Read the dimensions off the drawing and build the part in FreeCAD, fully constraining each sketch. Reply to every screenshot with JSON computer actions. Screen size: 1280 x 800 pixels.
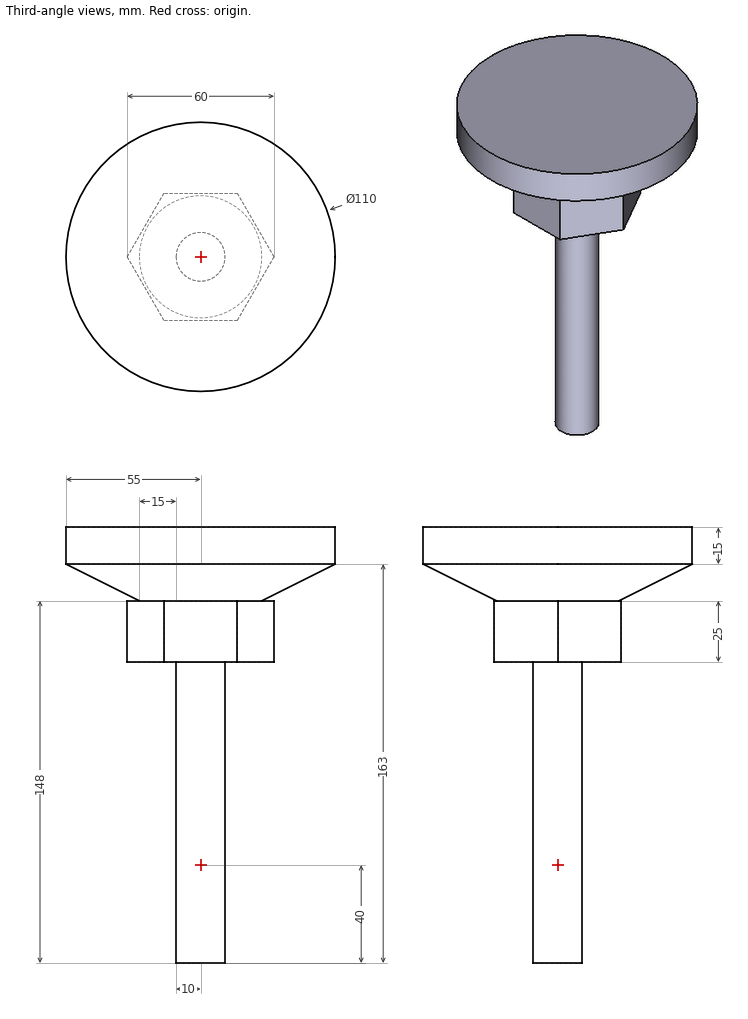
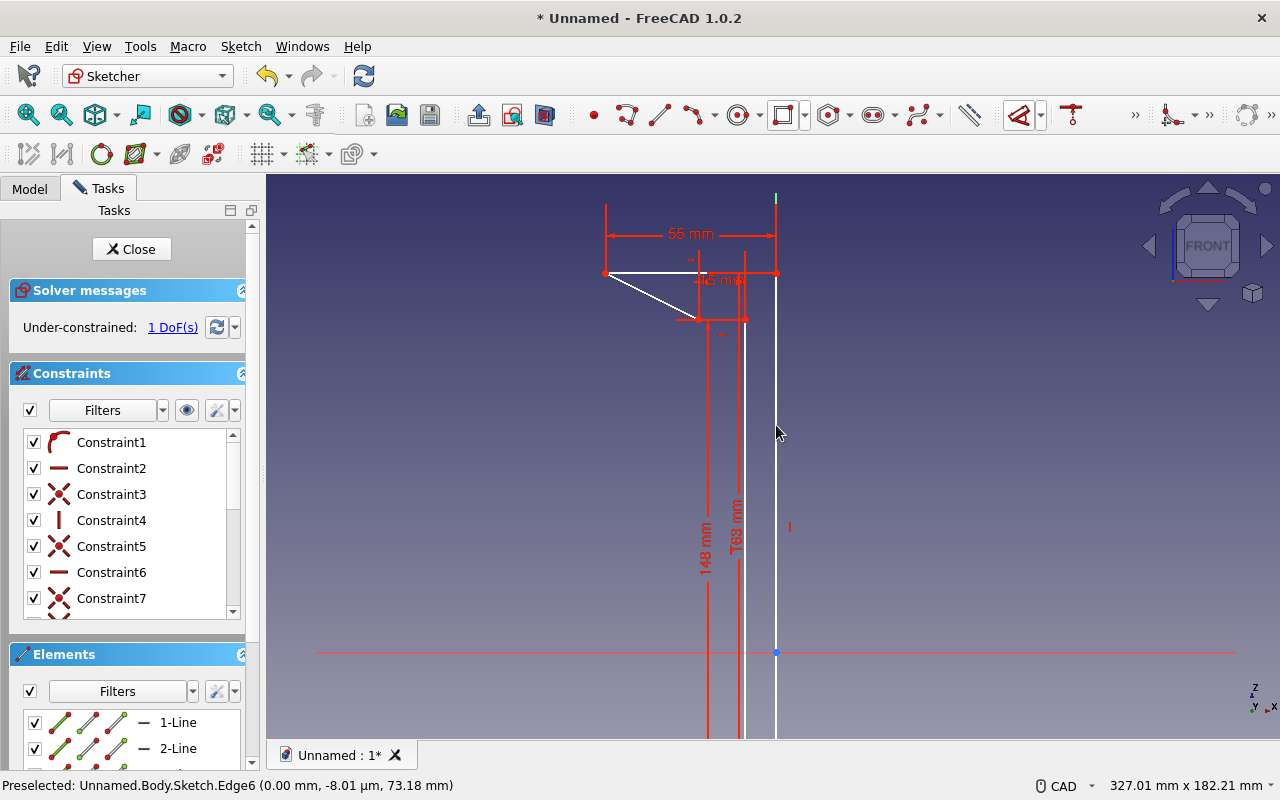
{"action": "scroll", "coordinate": [732, 319], "scroll_direction": "down", "scroll_amount": 2}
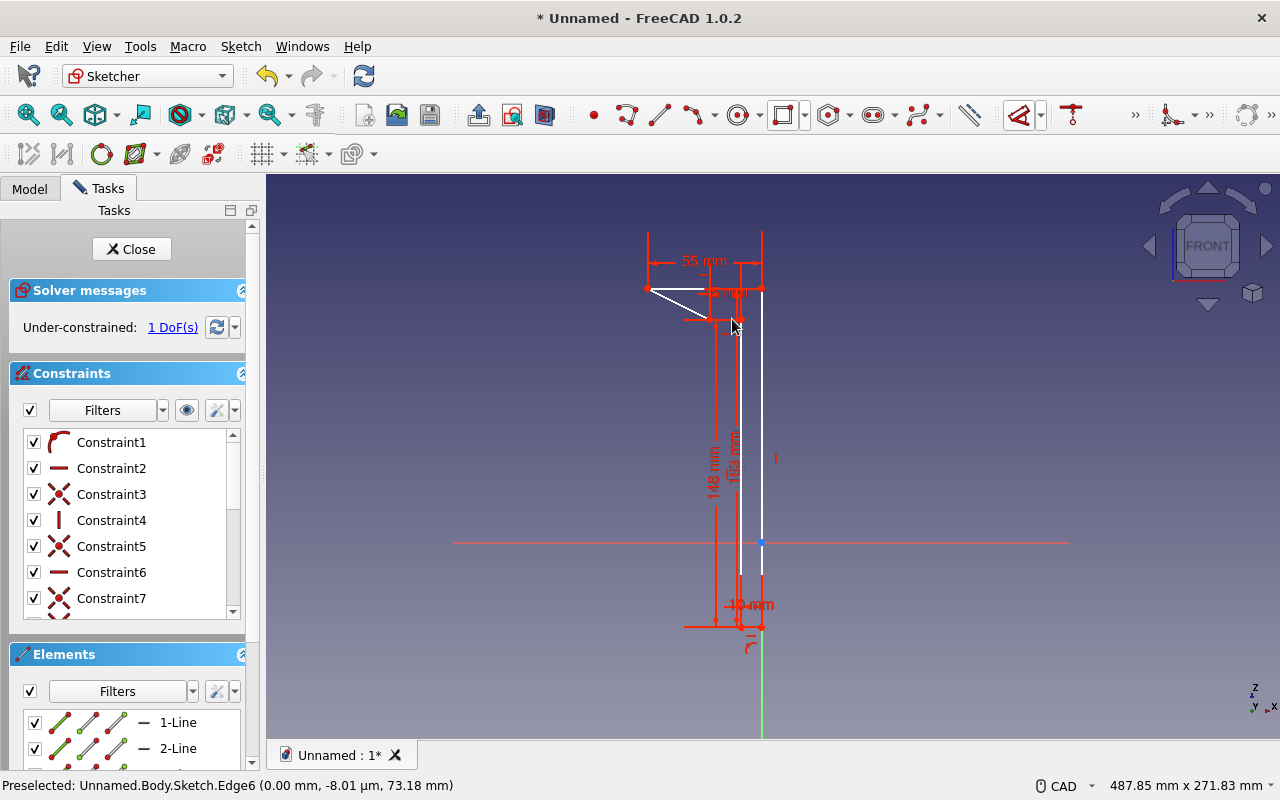
{"action": "left_click", "coordinate": [762, 627]}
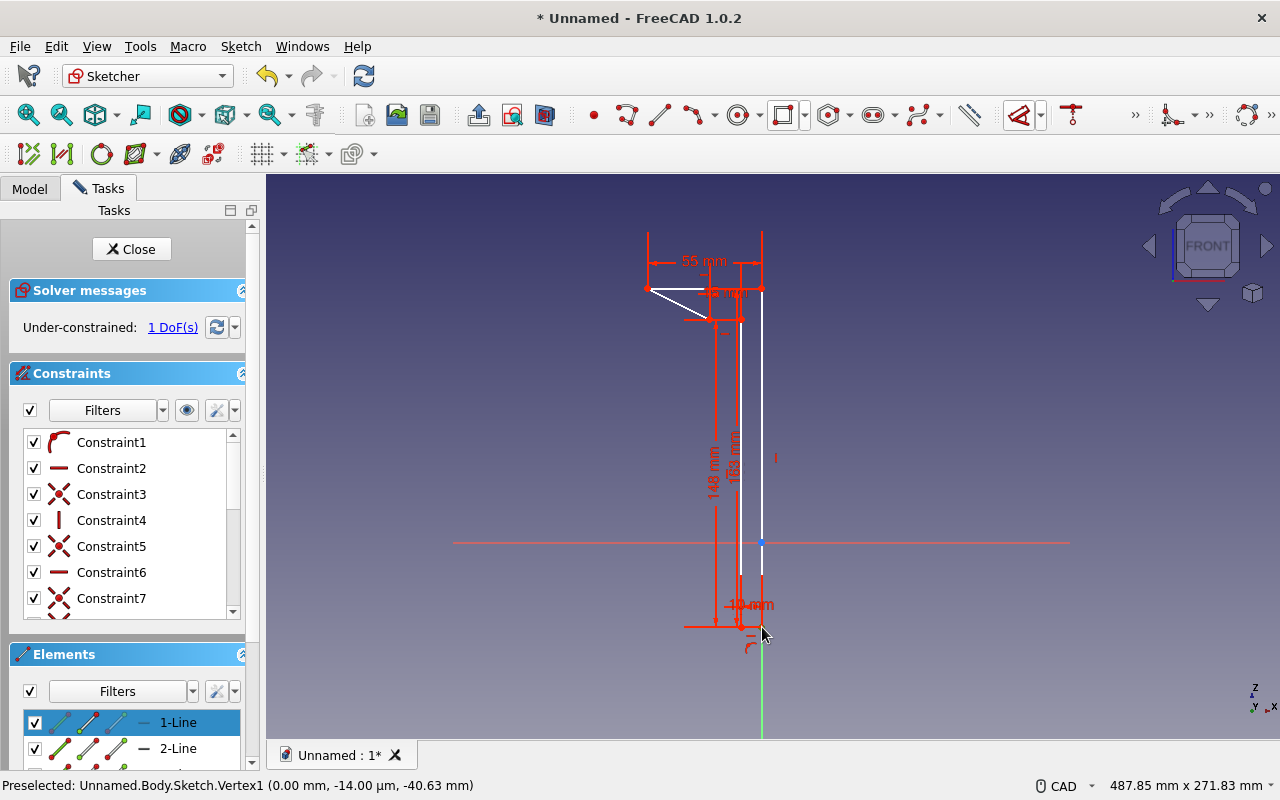
{"action": "key", "text": "i"}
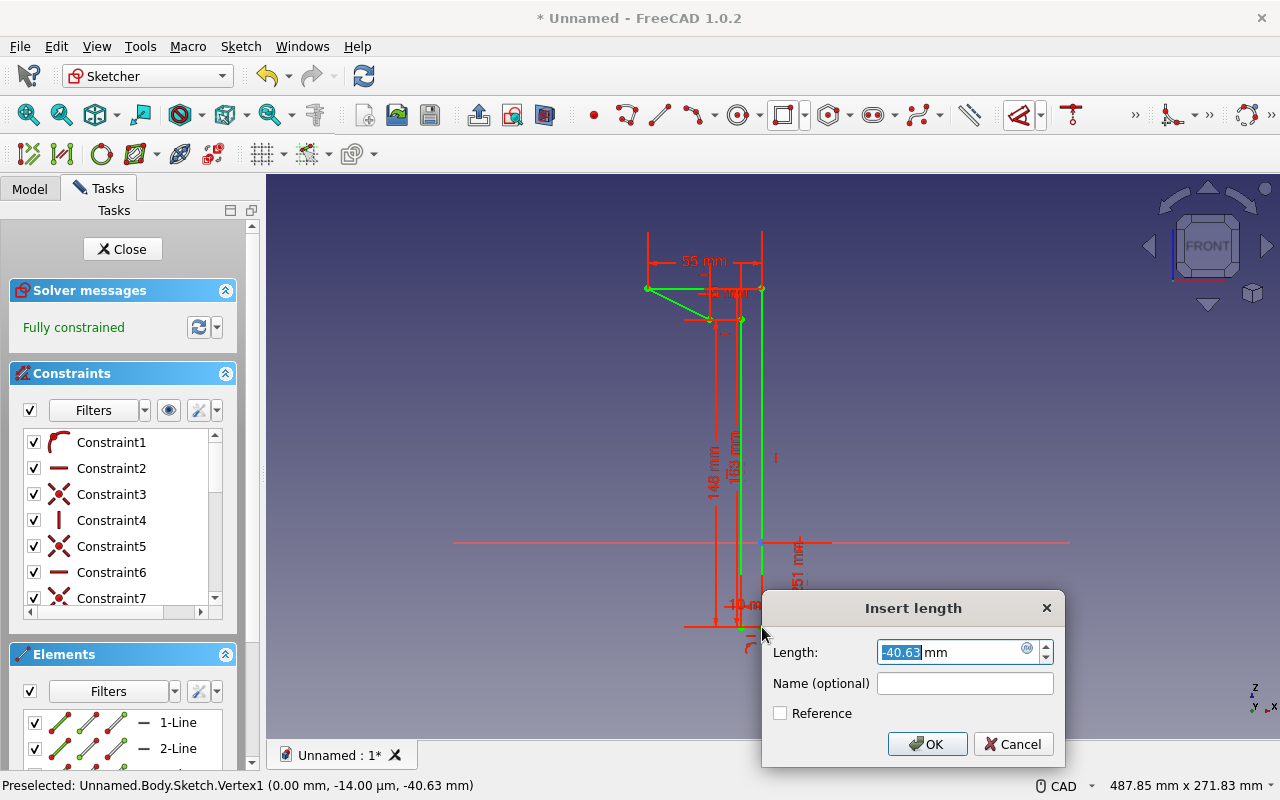
{"action": "type", "text": "-40"}
{"action": "key", "text": "Return"}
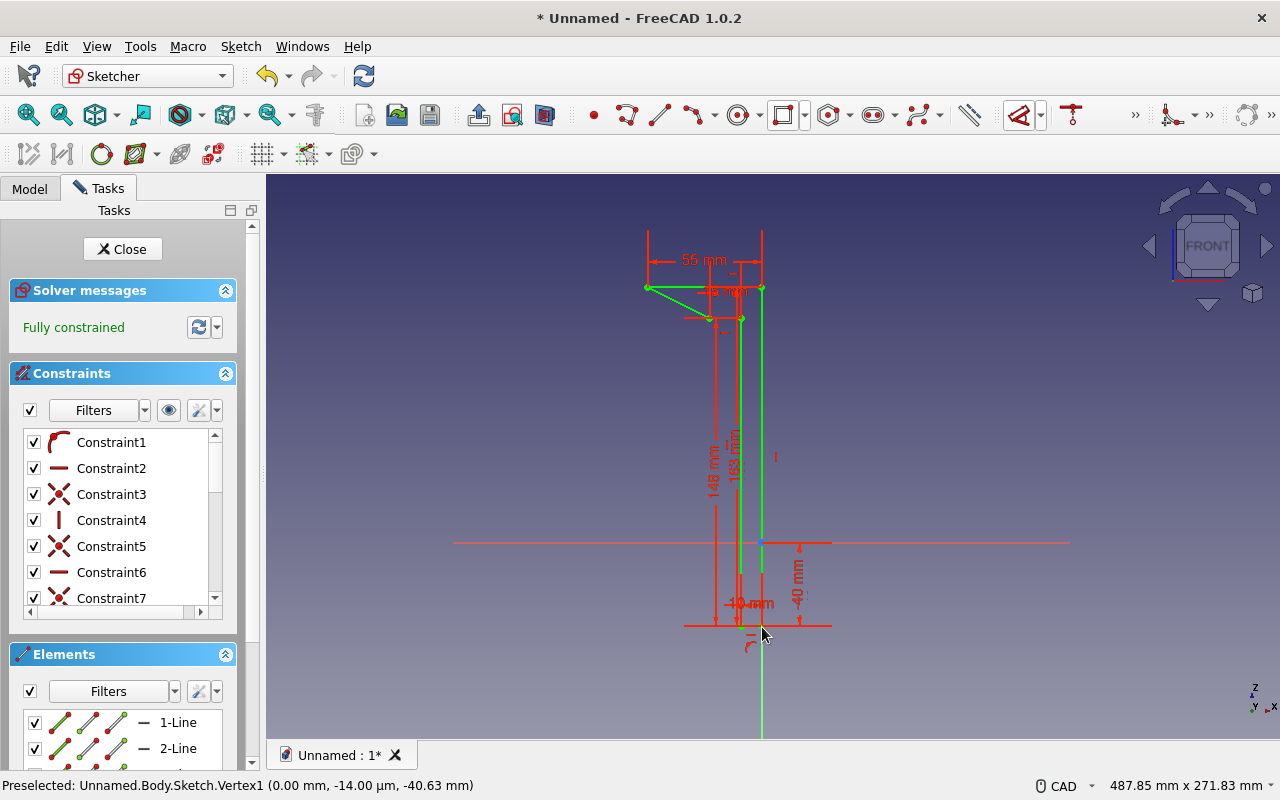
{"action": "left_click", "coordinate": [123, 249]}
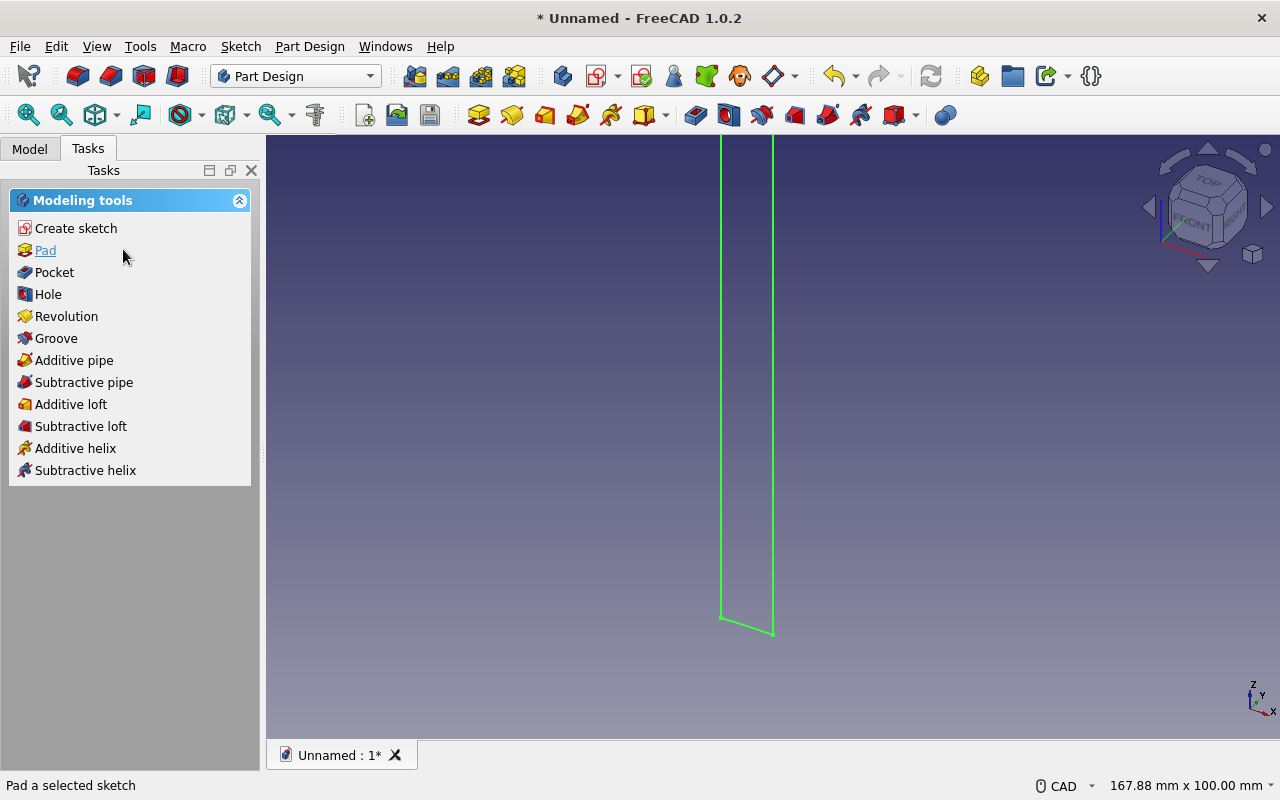
{"action": "left_click", "coordinate": [512, 116]}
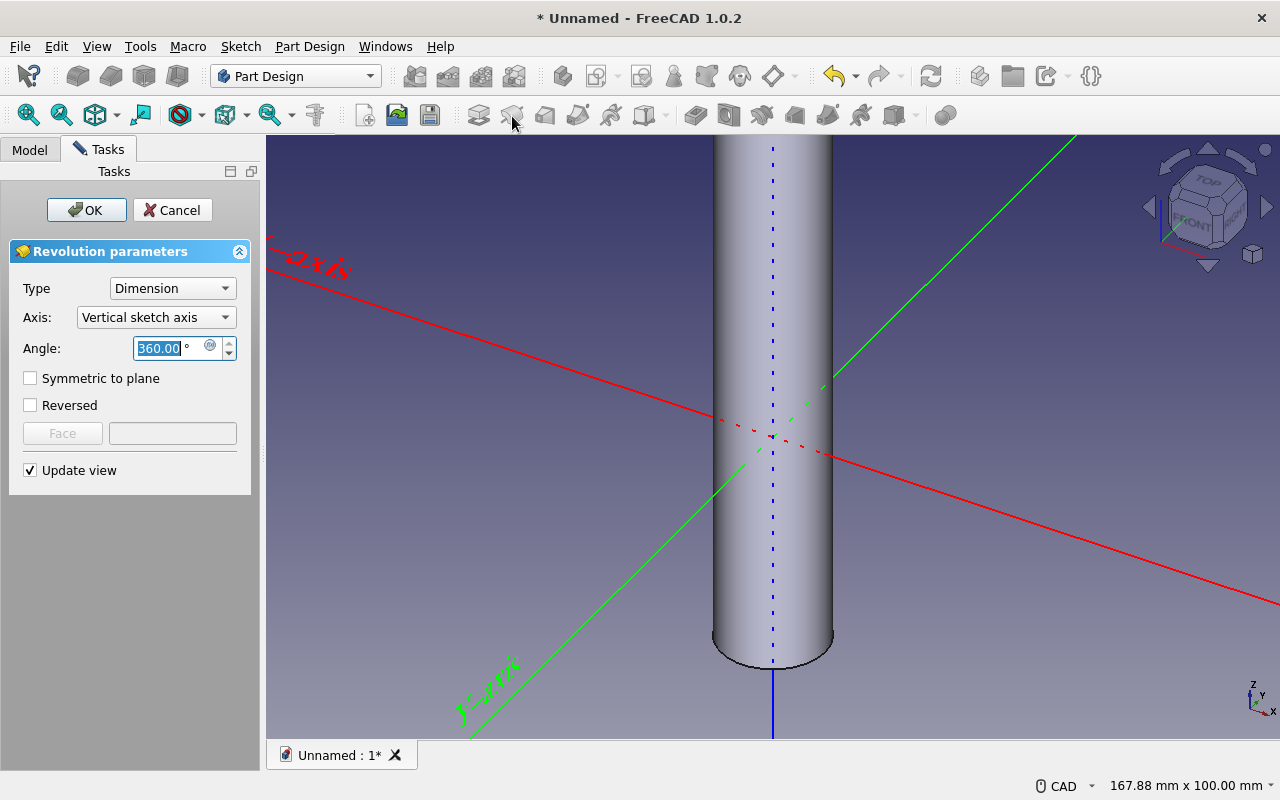
{"action": "left_click", "coordinate": [87, 210]}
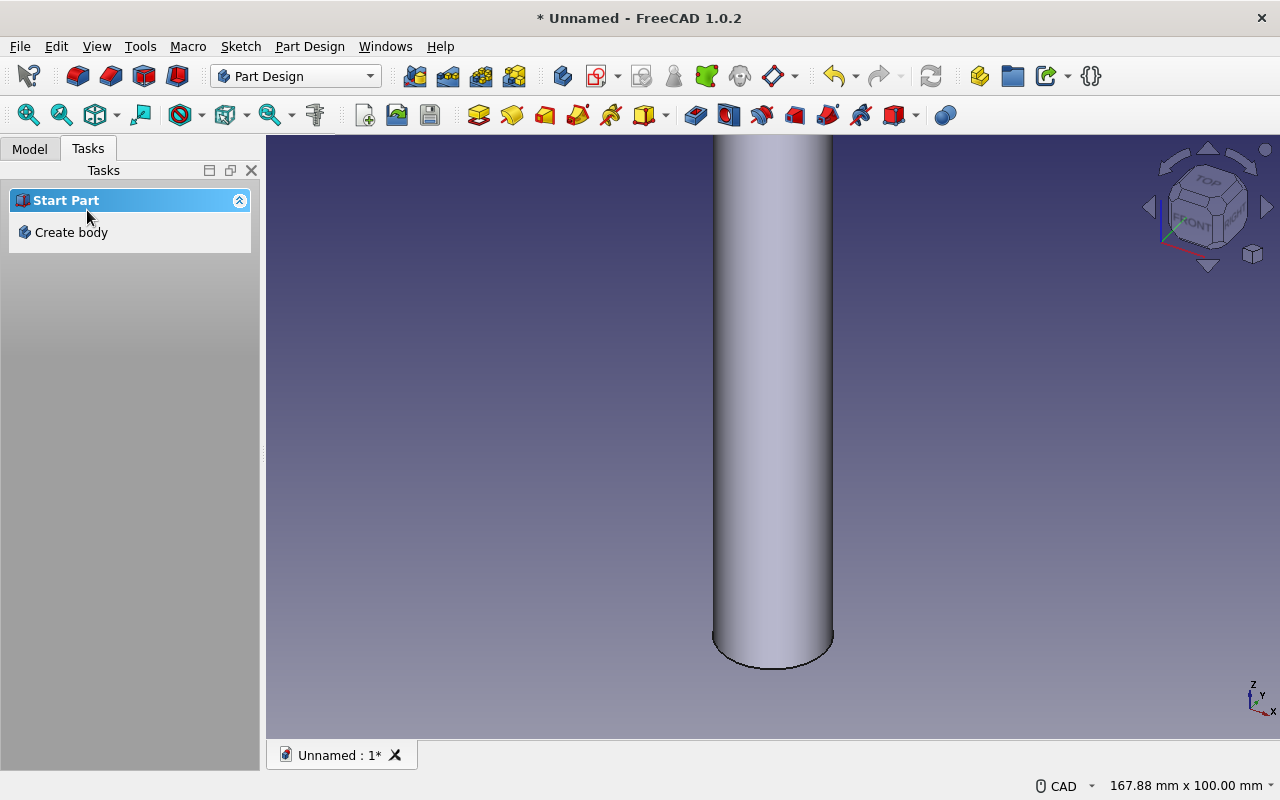
{"action": "left_click", "coordinate": [29, 116]}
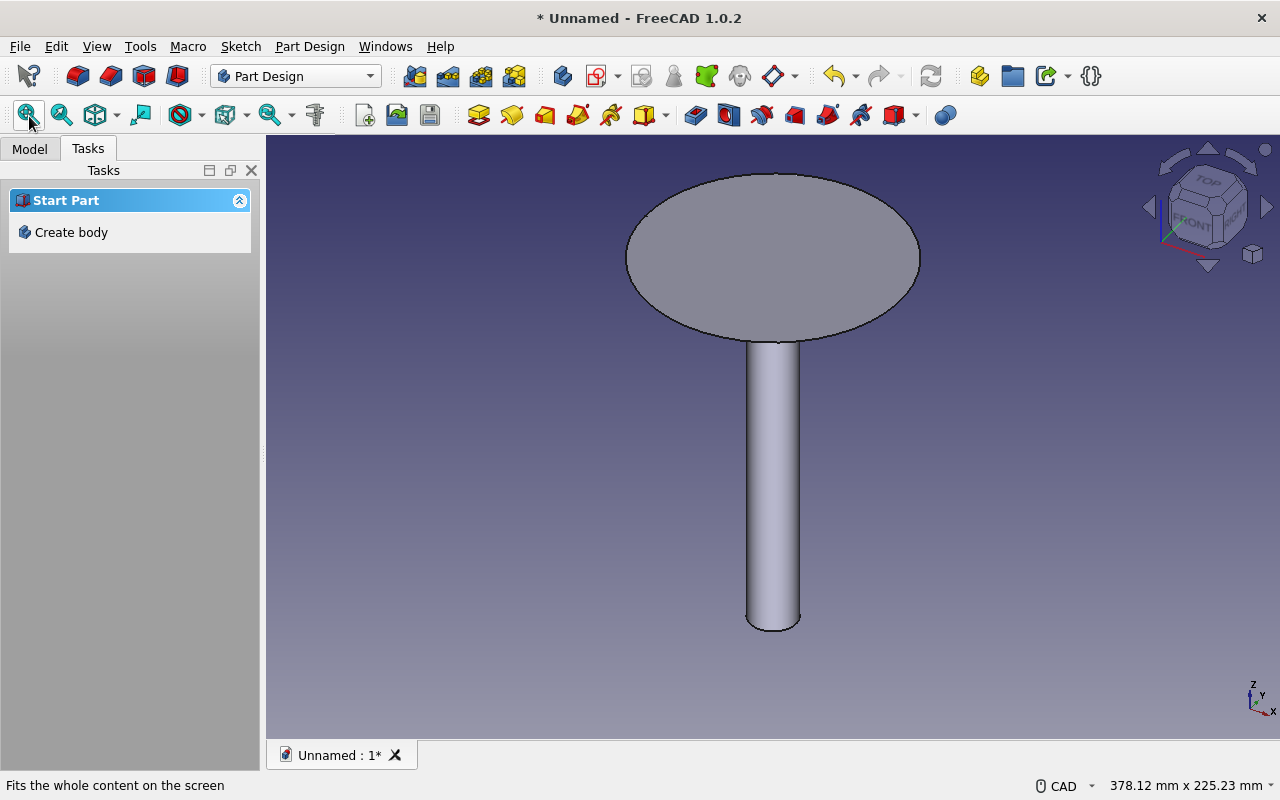
{"action": "left_click", "coordinate": [773, 257]}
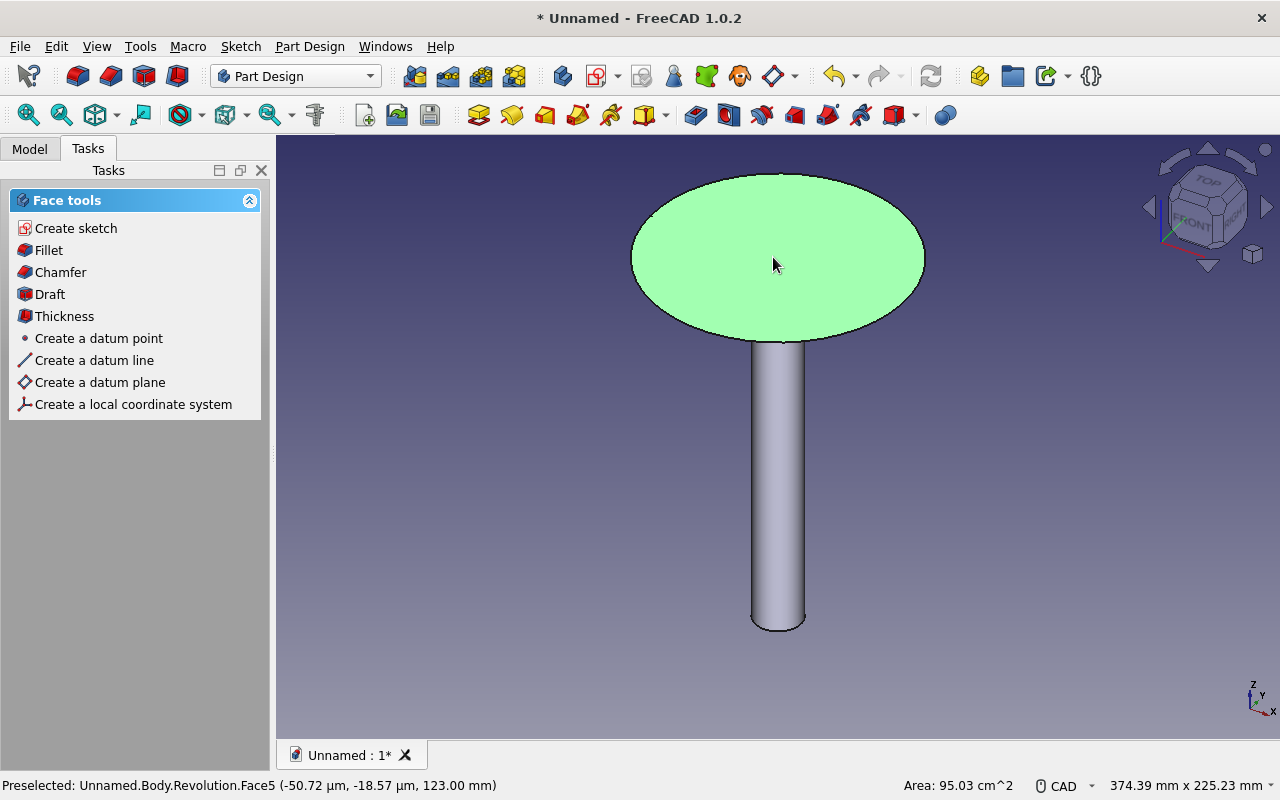
{"action": "left_click", "coordinate": [596, 76]}